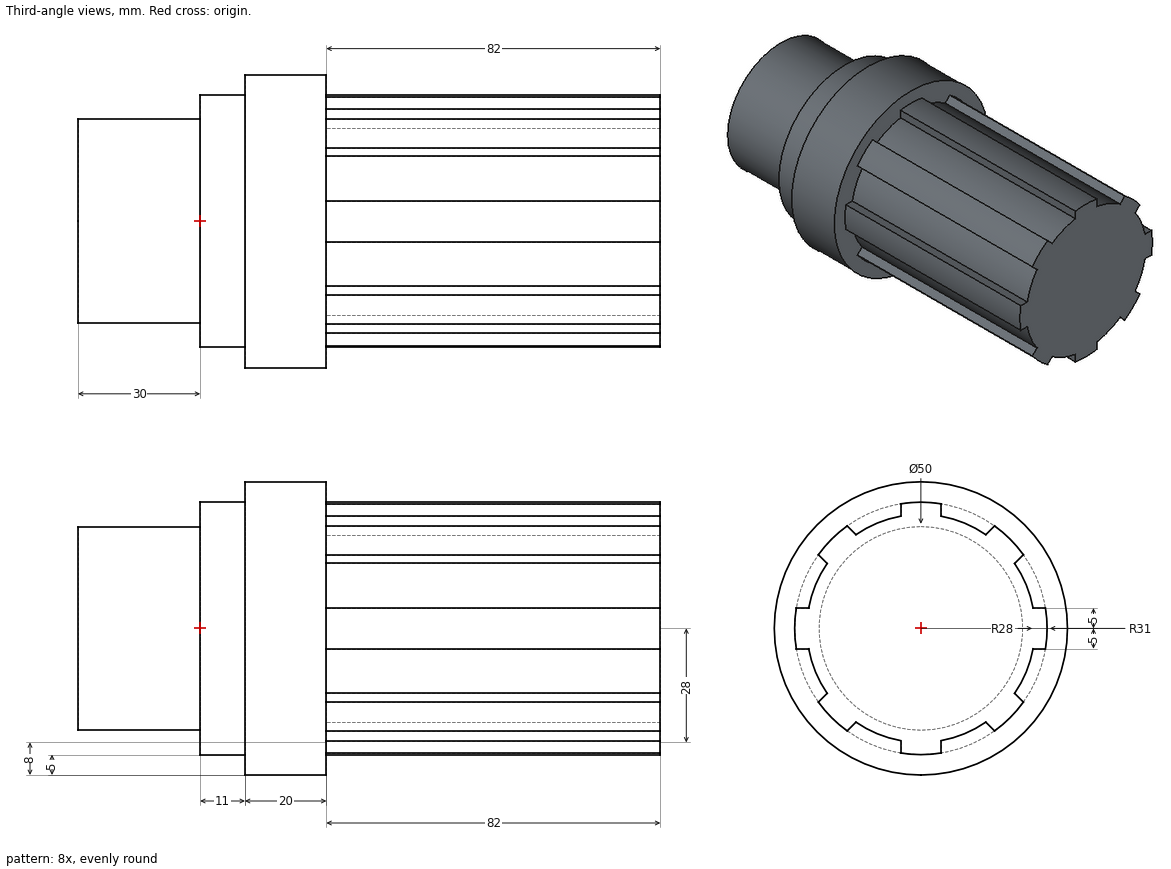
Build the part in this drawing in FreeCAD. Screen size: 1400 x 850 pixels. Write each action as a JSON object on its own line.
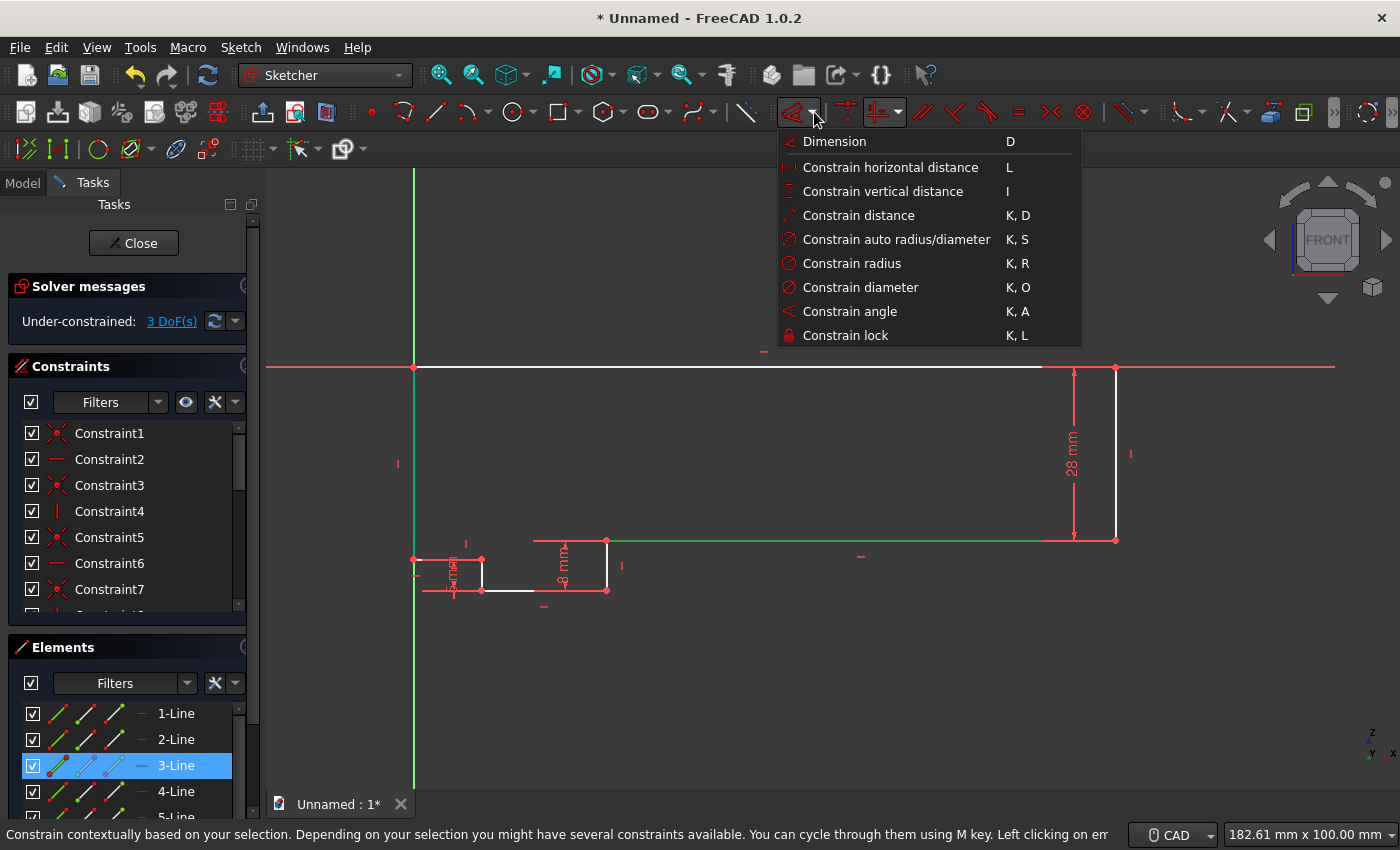
{"action": "left_click", "coordinate": [930, 167]}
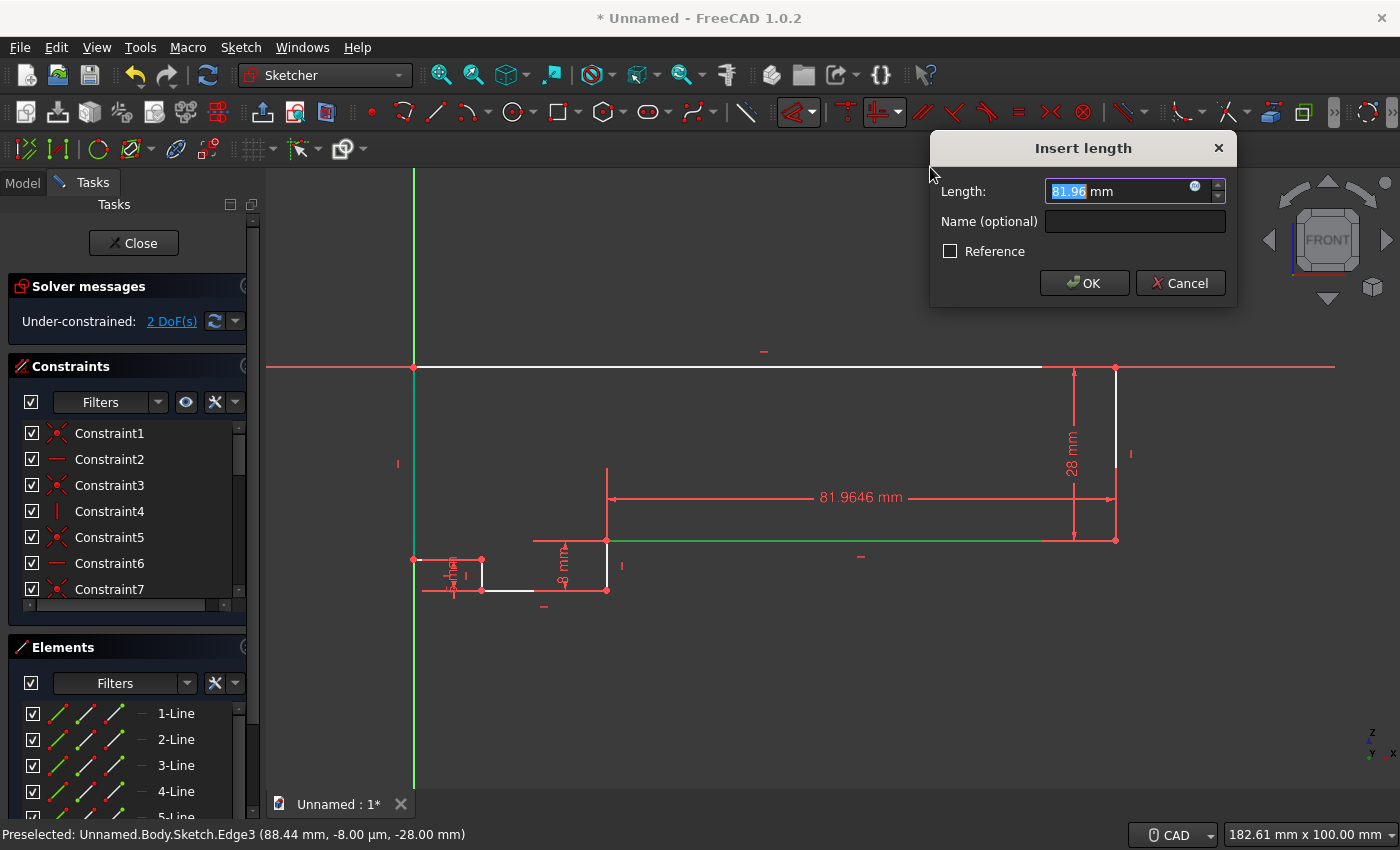
{"action": "type", "text": "82"}
{"action": "key", "text": "Return"}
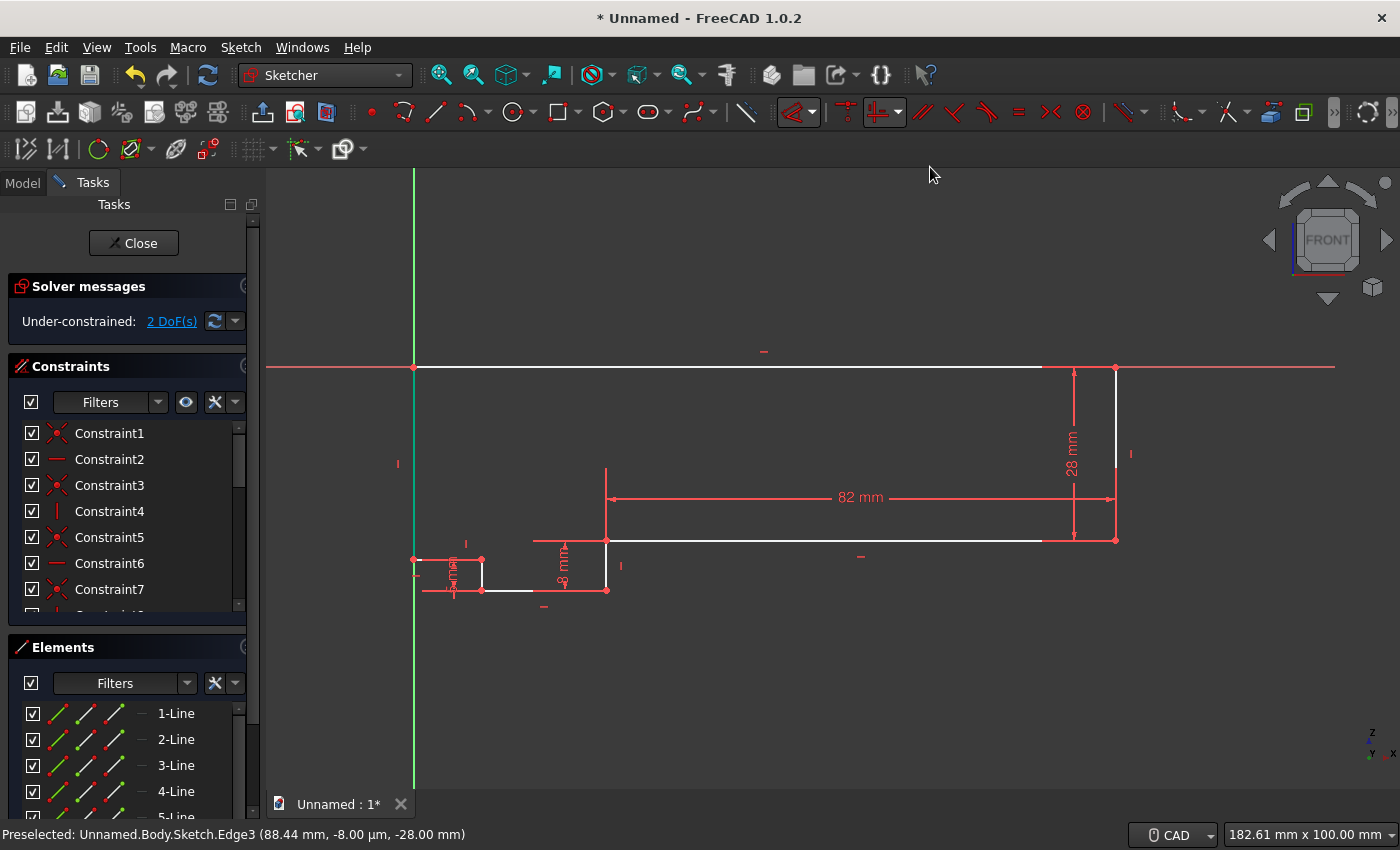
{"action": "left_click", "coordinate": [569, 591]}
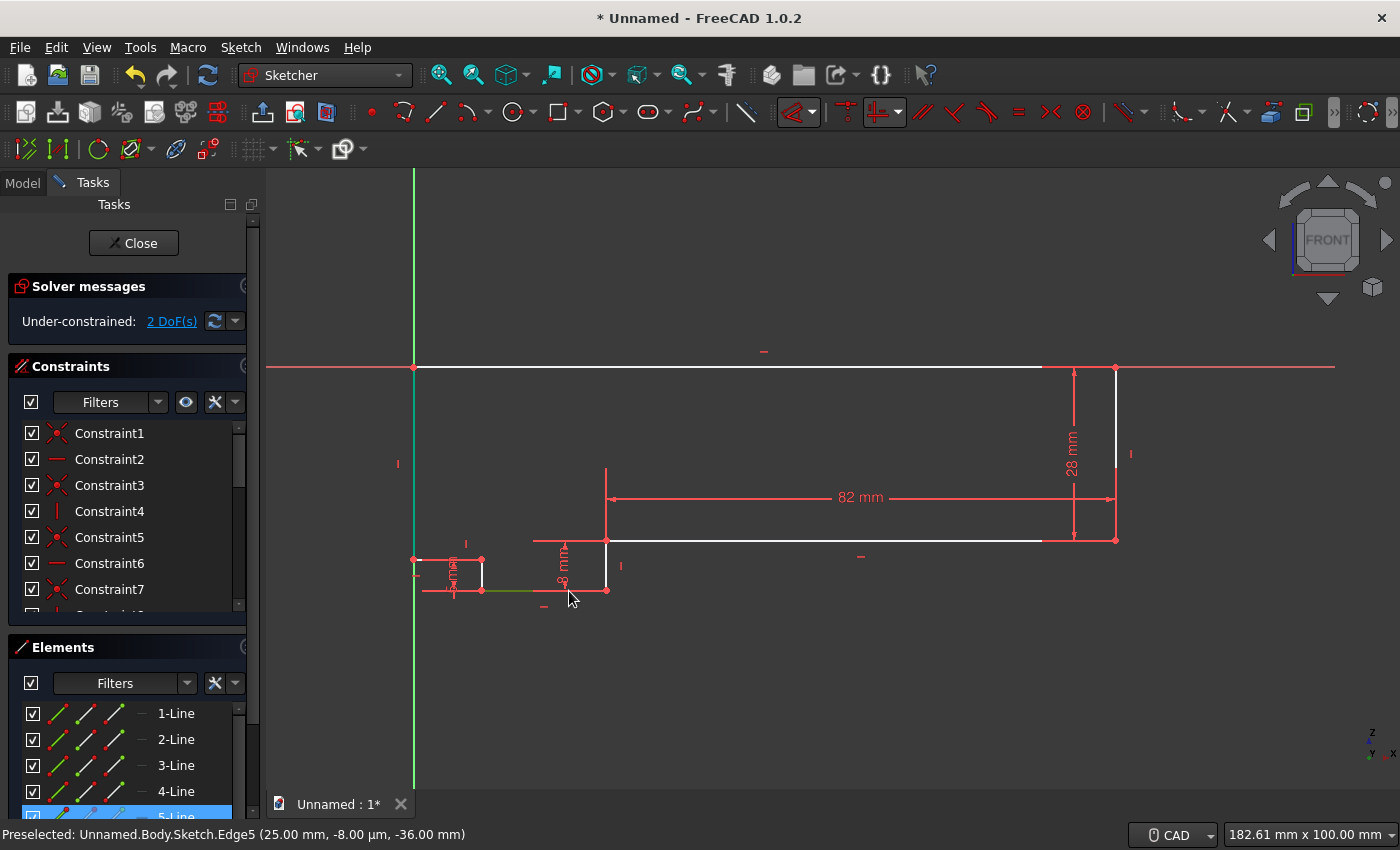
{"action": "key", "text": "l"}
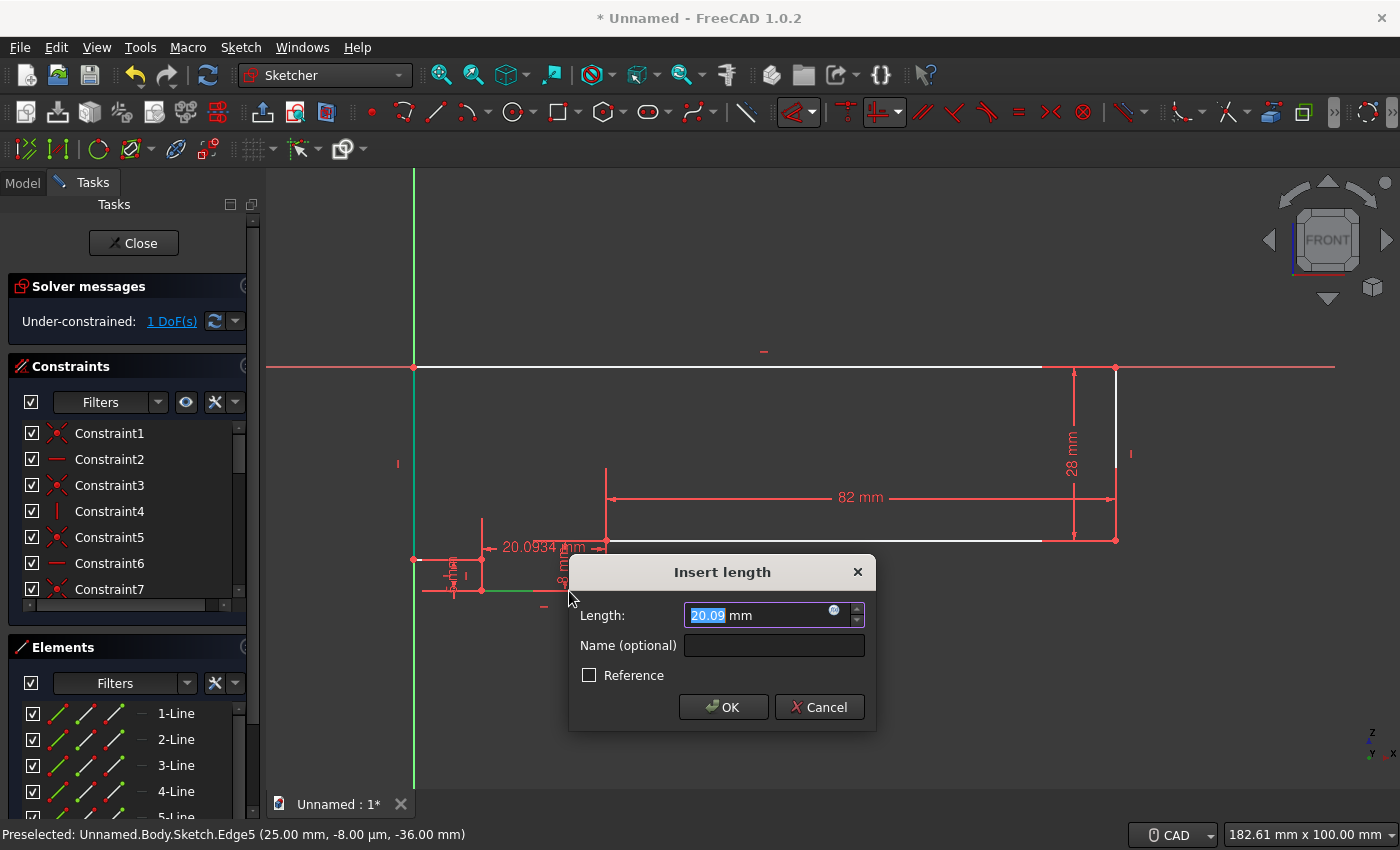
{"action": "type", "text": "20"}
{"action": "key", "text": "Return"}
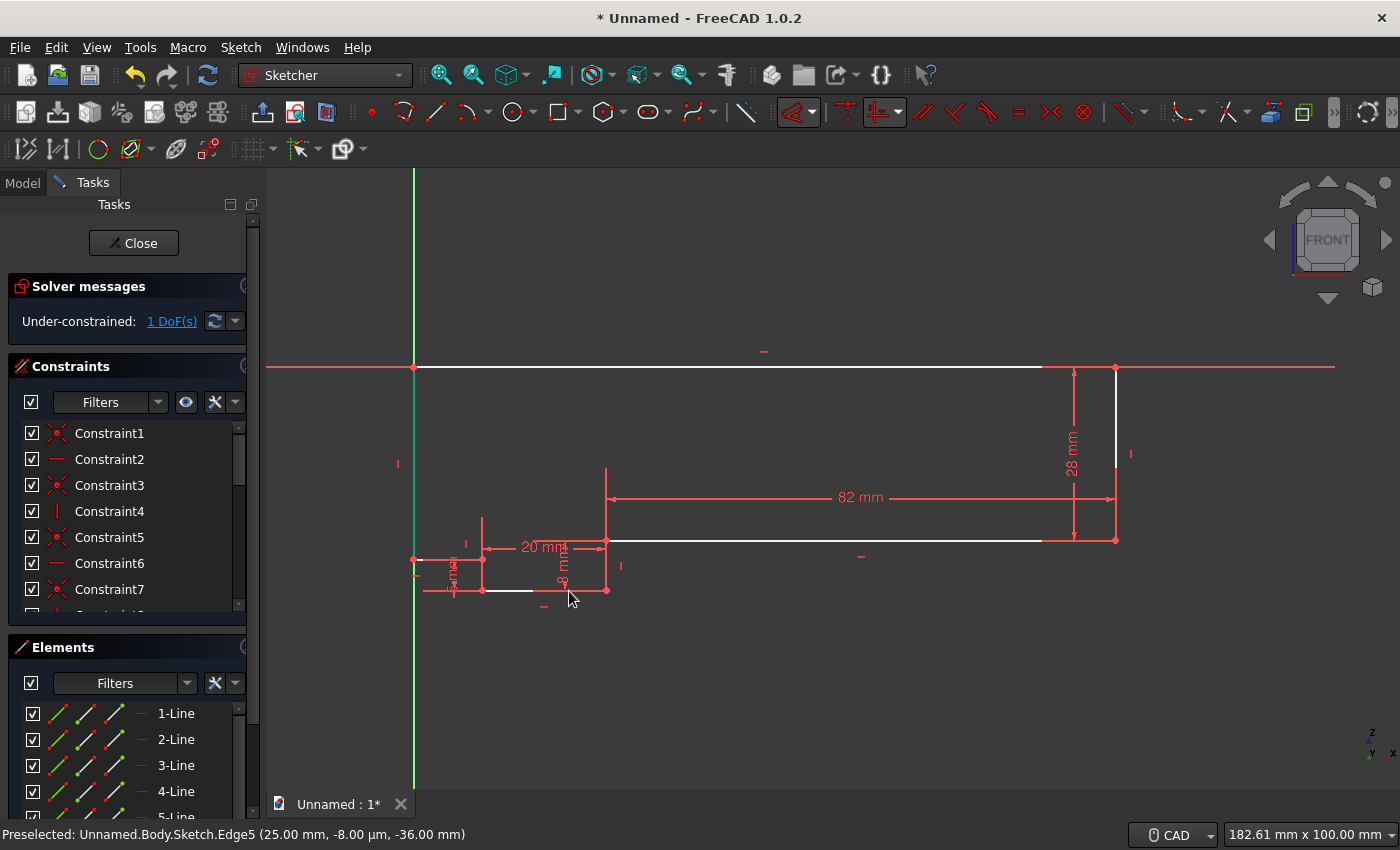
{"action": "left_click", "coordinate": [434, 560]}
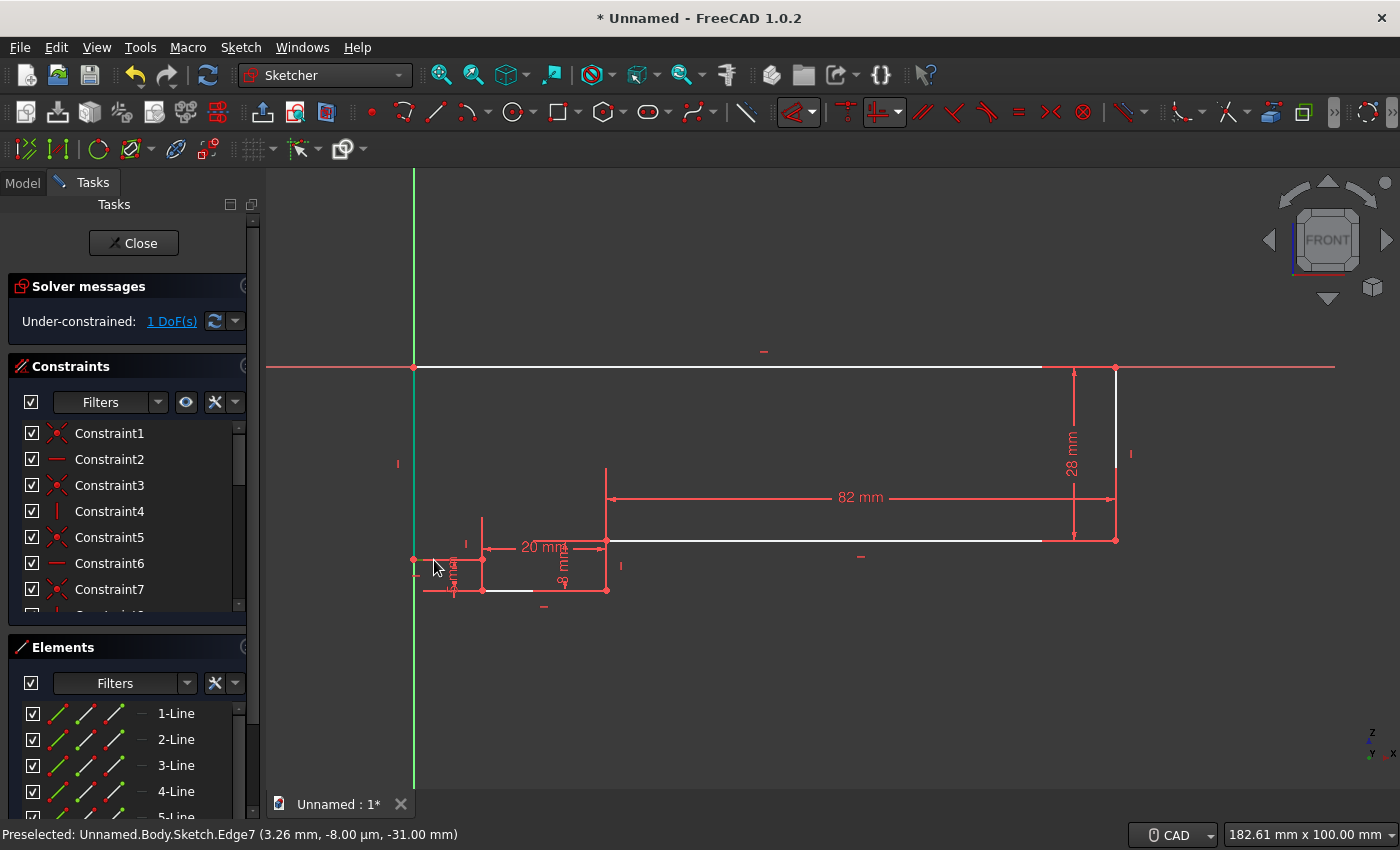
{"action": "key", "text": "l"}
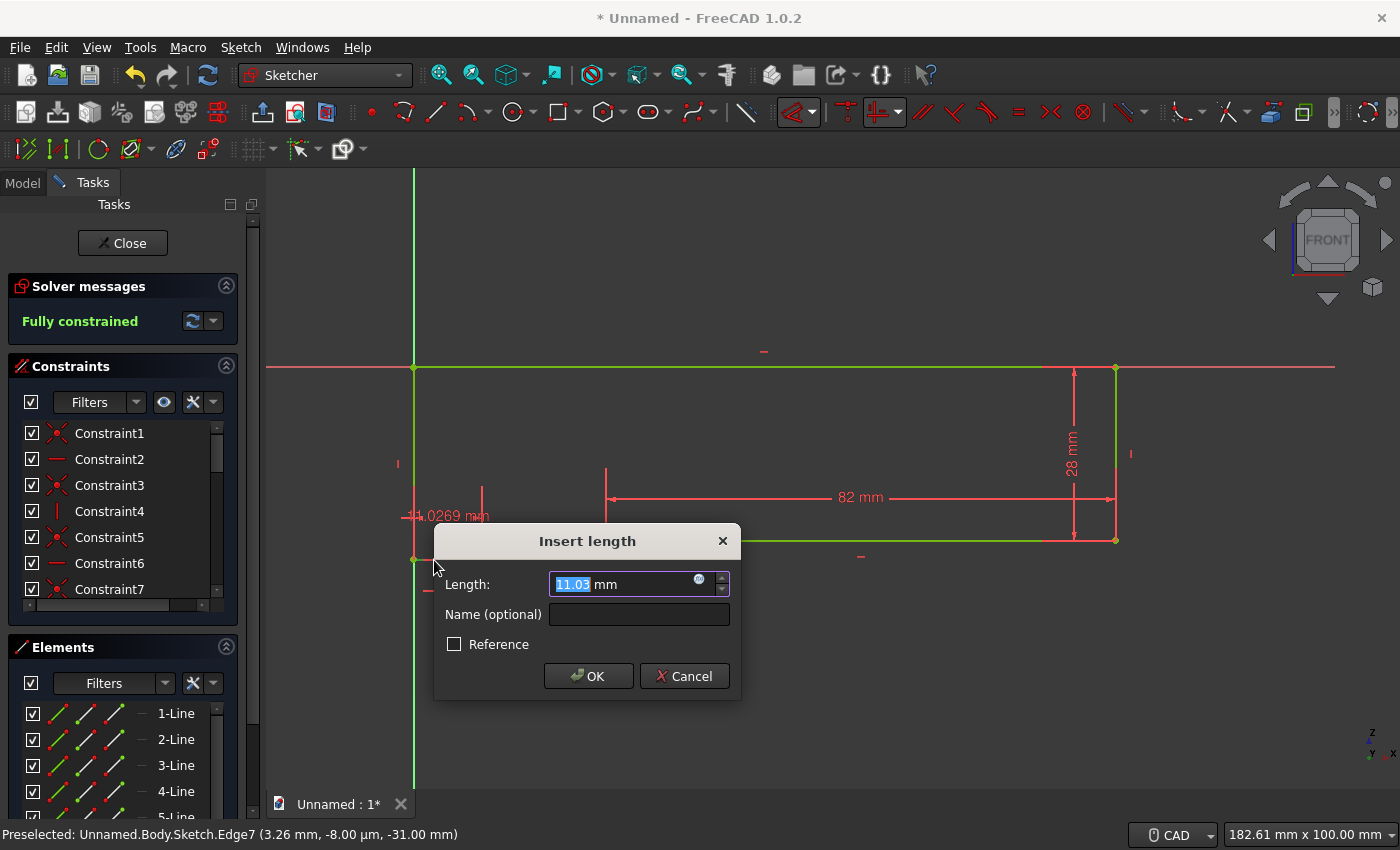
{"action": "type", "text": "11"}
{"action": "key", "text": "Return"}